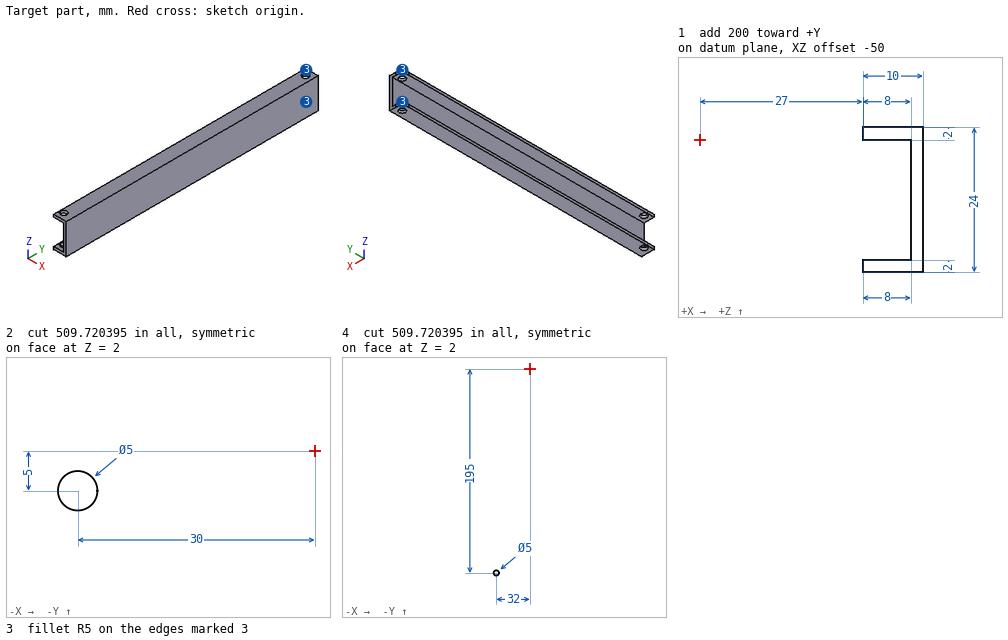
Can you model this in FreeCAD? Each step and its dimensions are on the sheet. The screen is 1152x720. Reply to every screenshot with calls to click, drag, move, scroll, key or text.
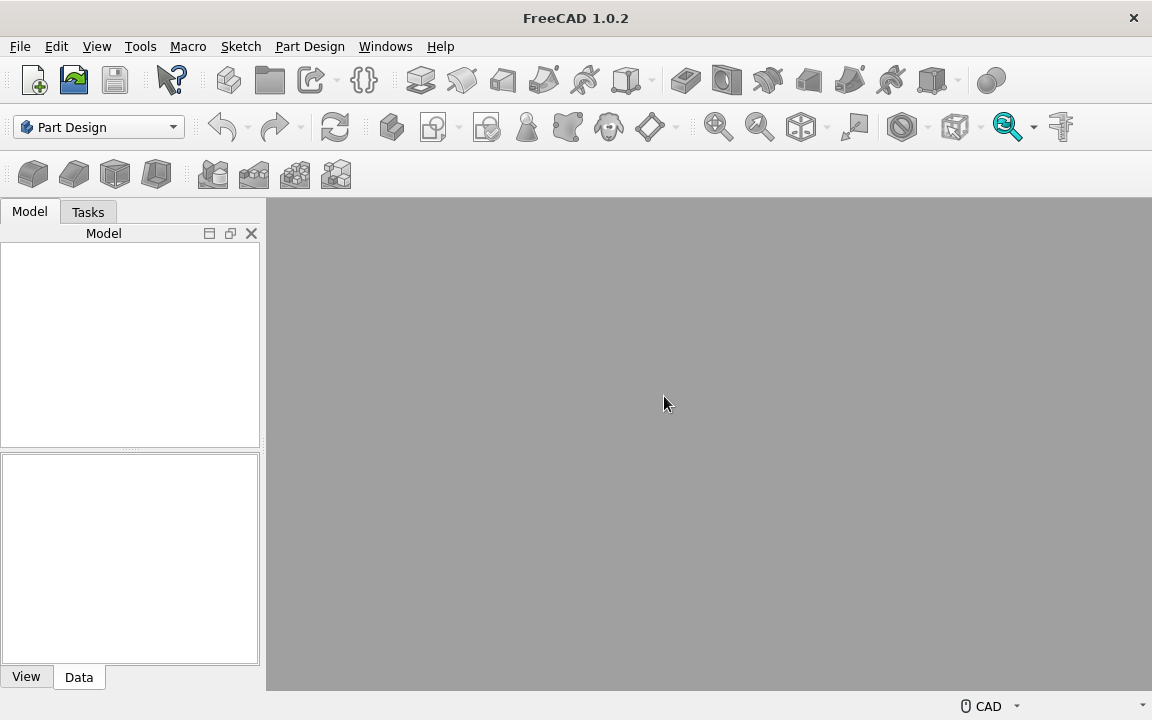
click(33, 80)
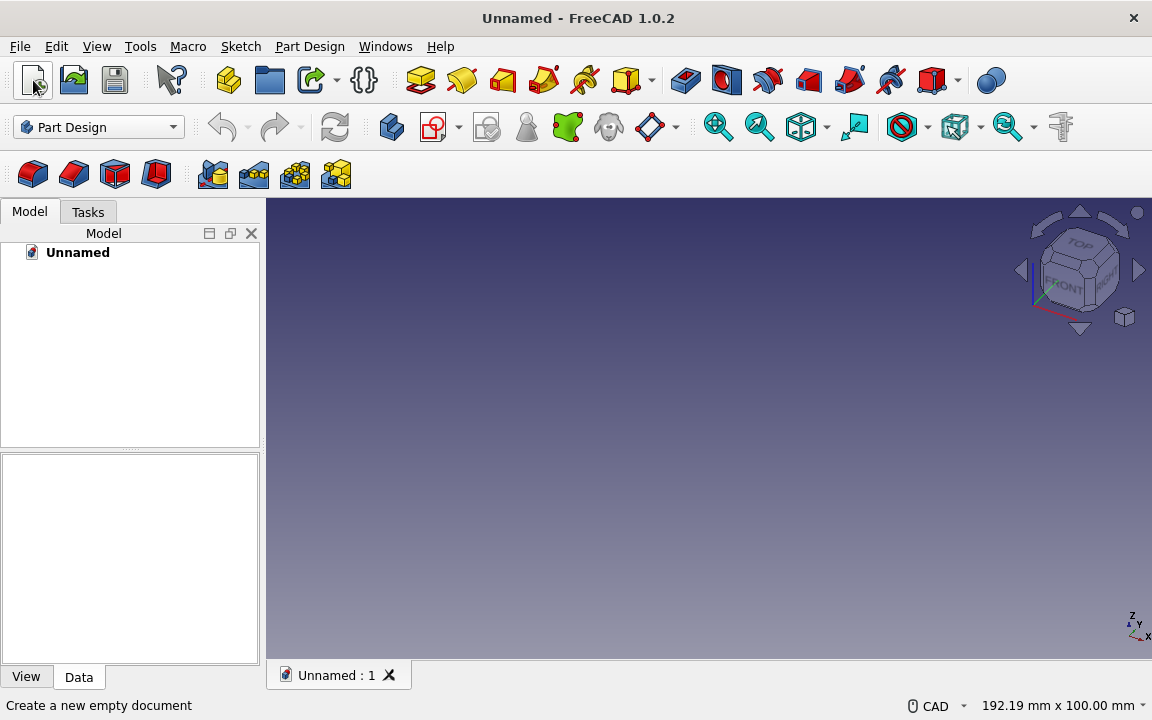
click(392, 128)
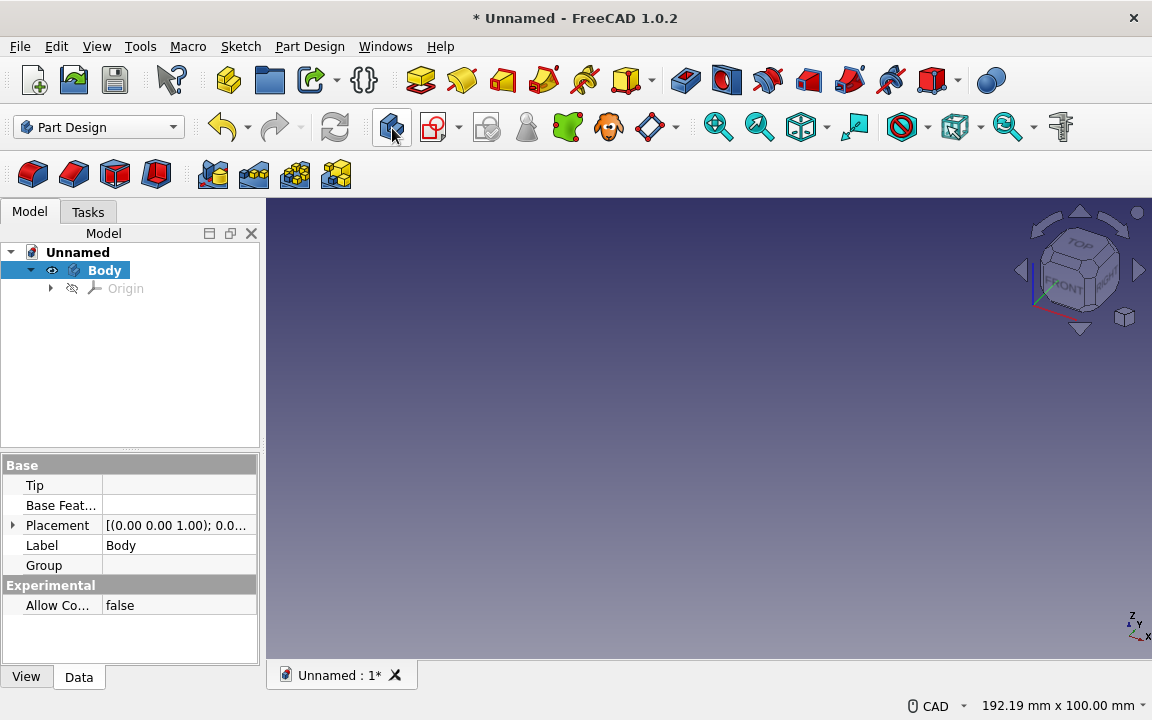
click(51, 288)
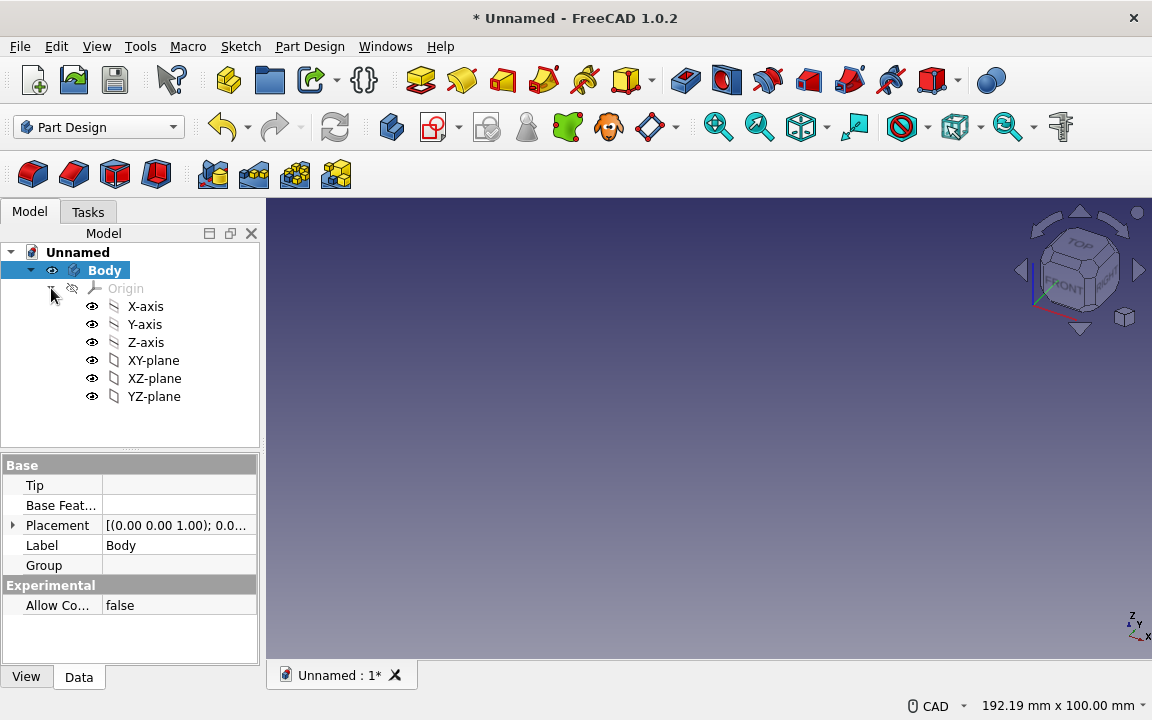
click(137, 378)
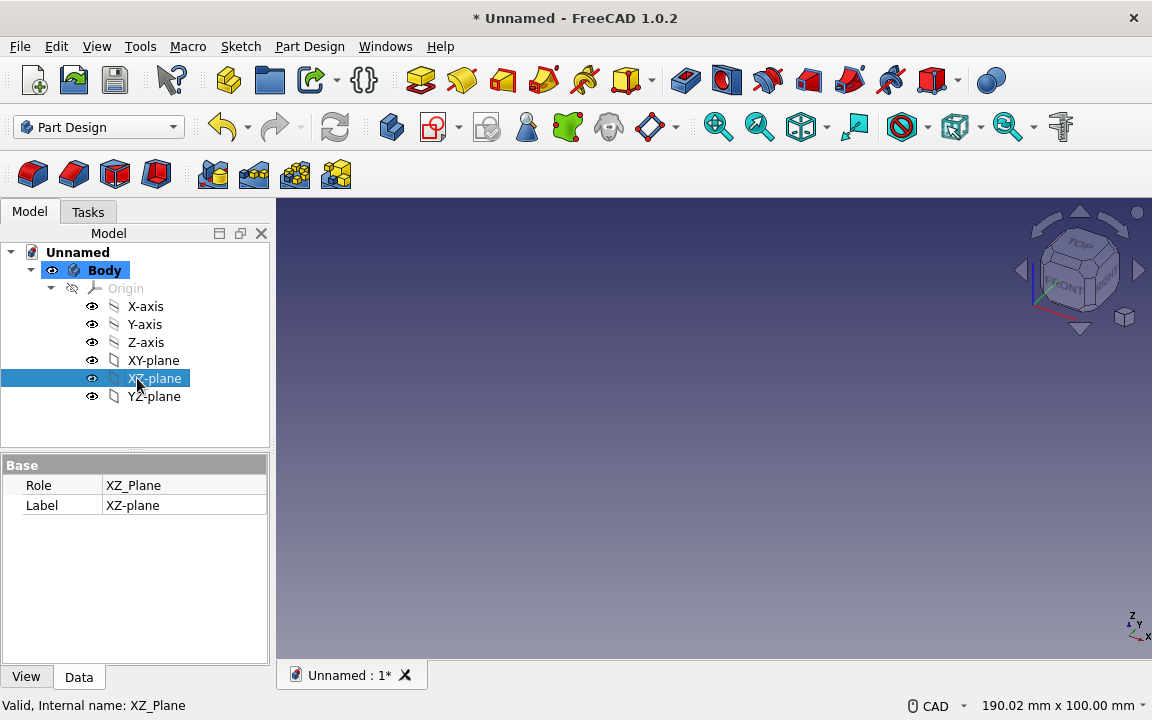
click(650, 128)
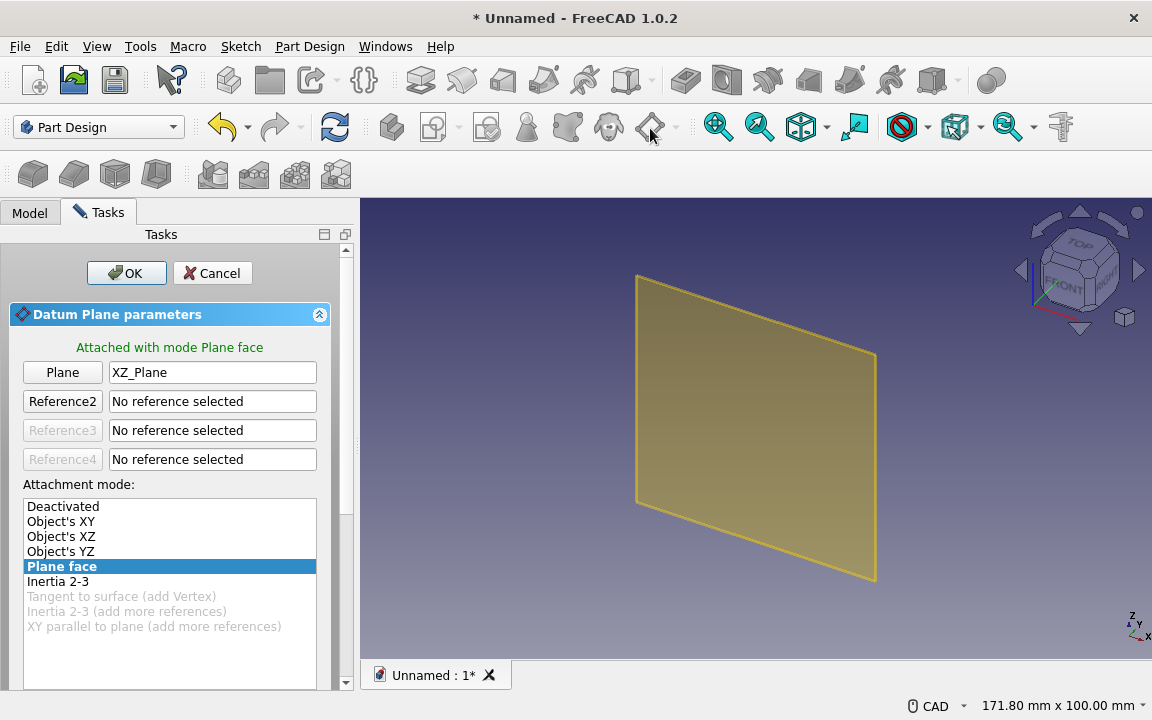
scroll(346, 467, down, 4)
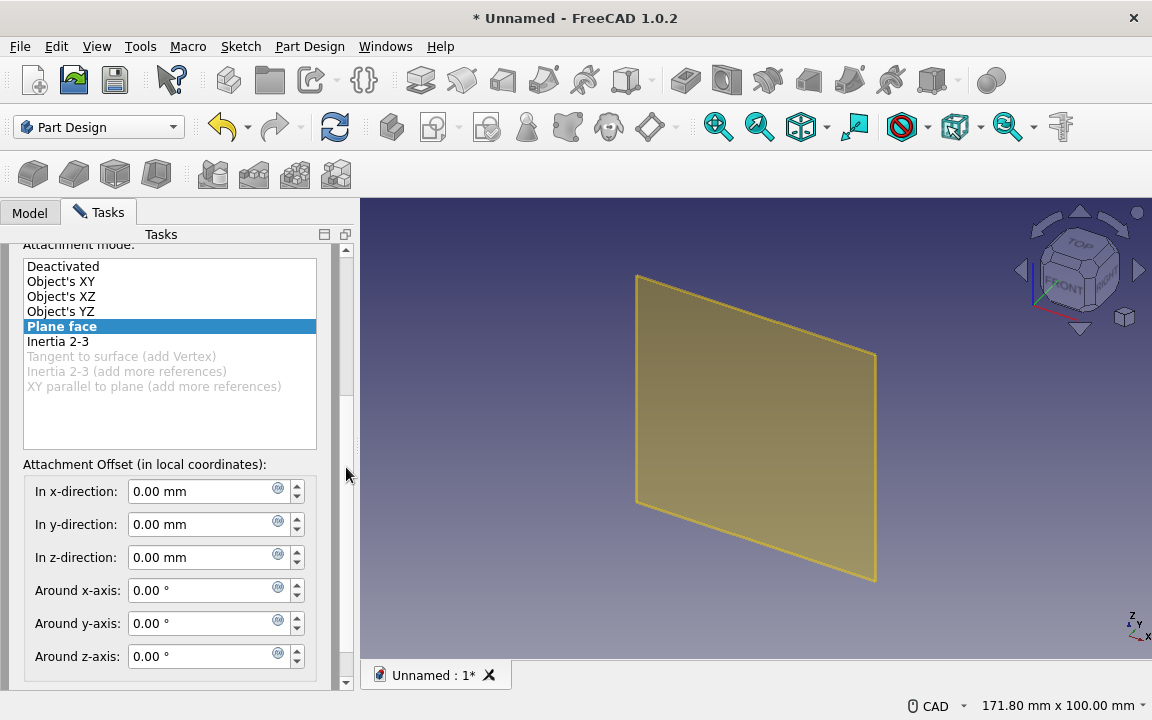
triple_click(210, 558)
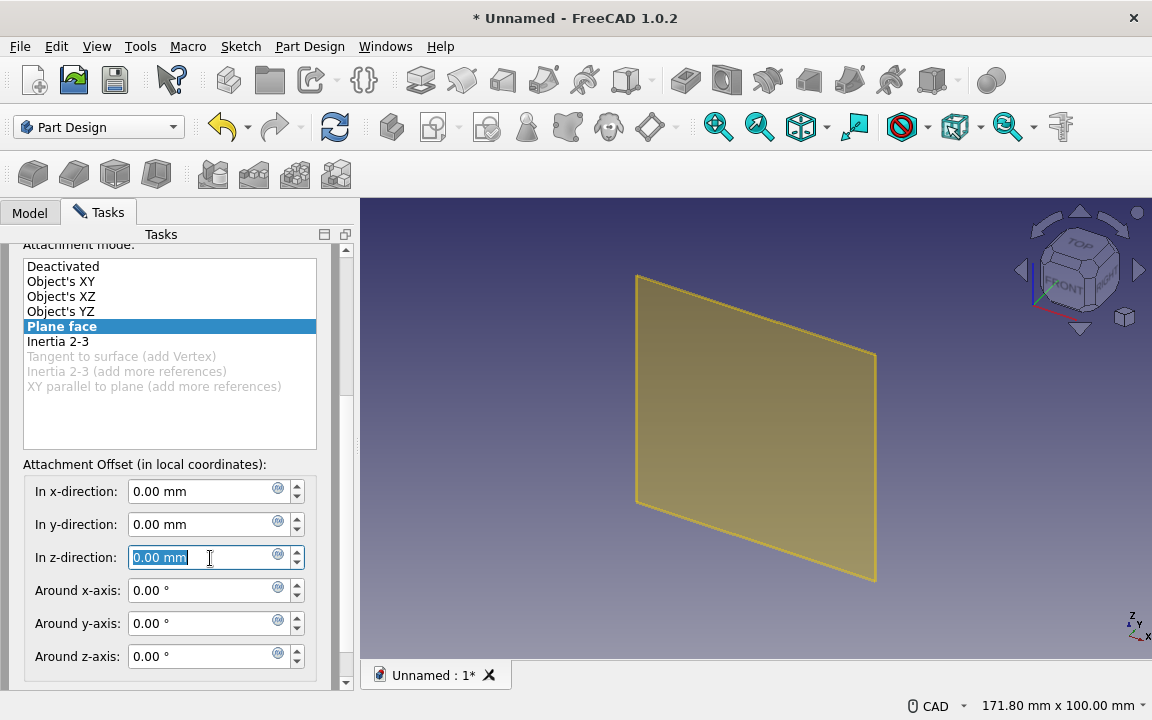
text(-50)
key(Tab)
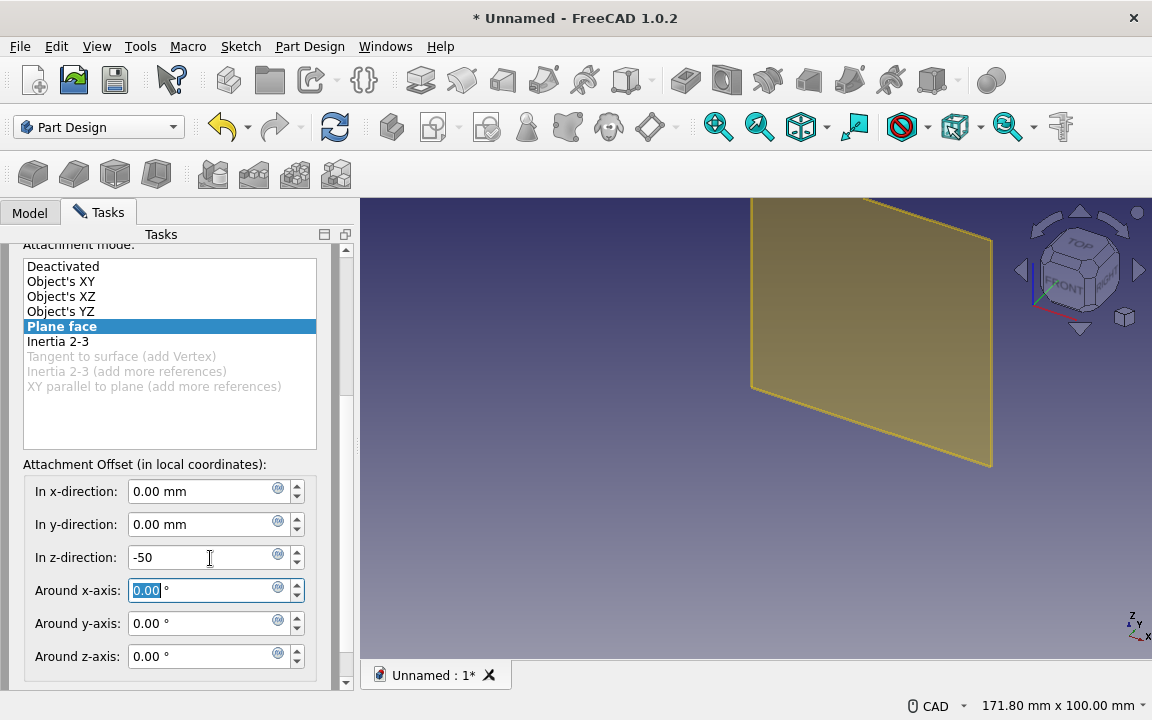
scroll(346, 467, up, 5)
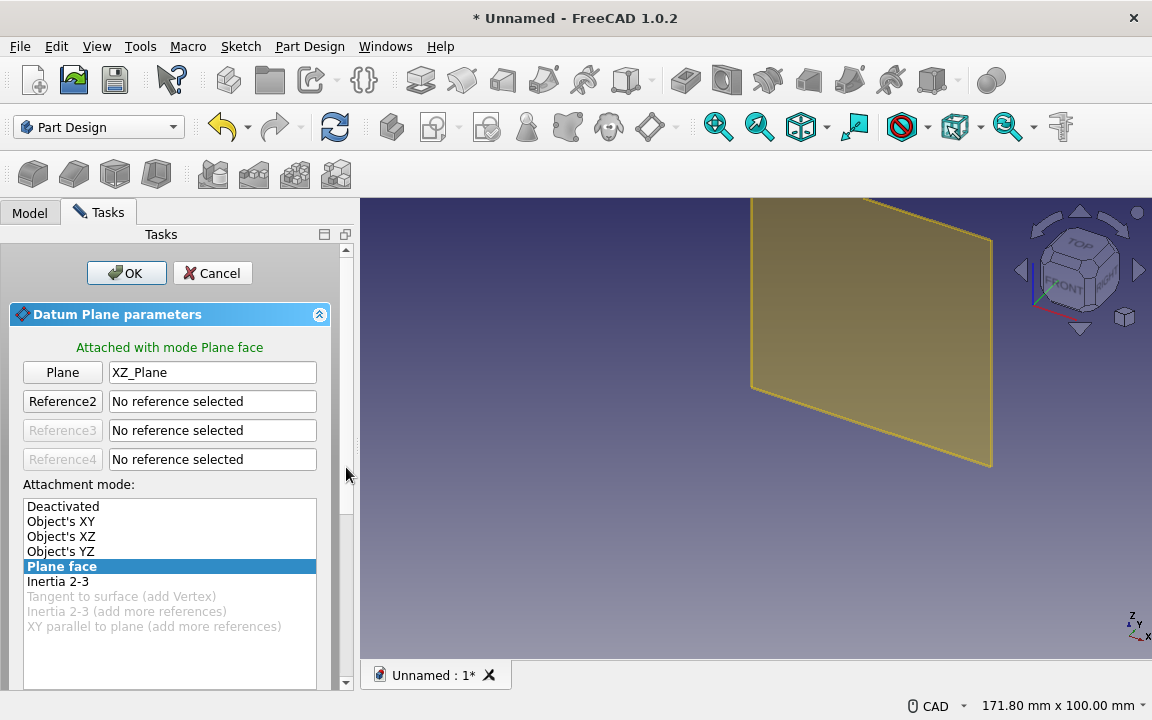
click(127, 273)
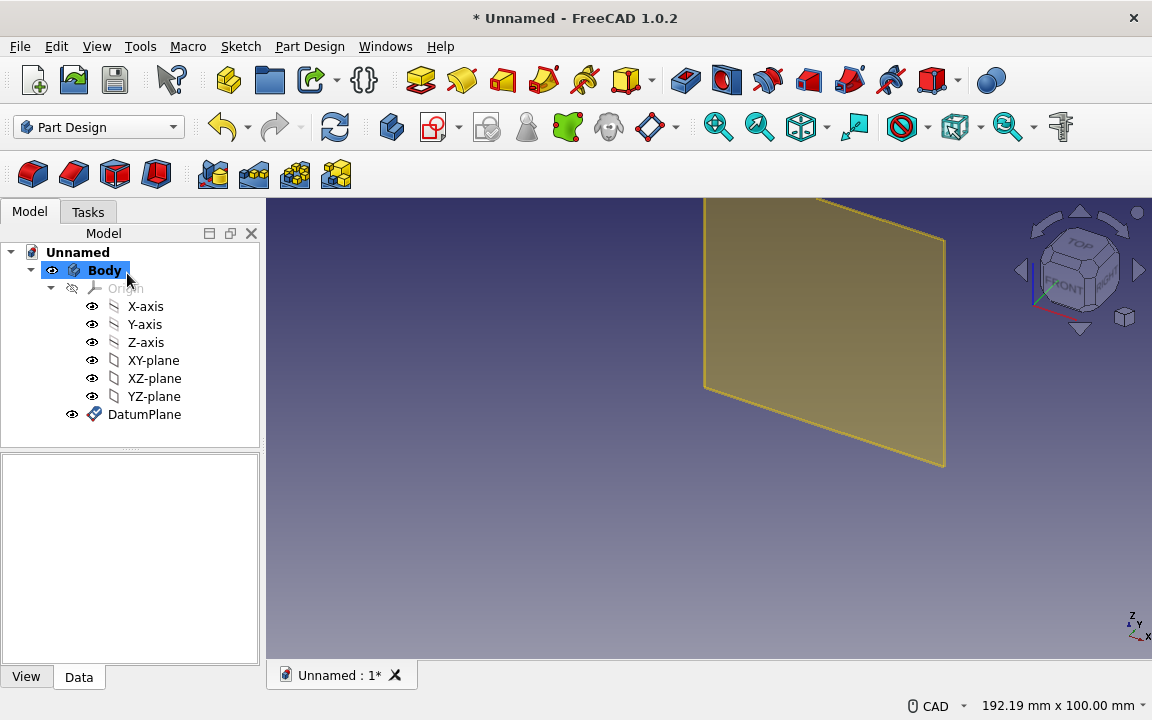
click(117, 414)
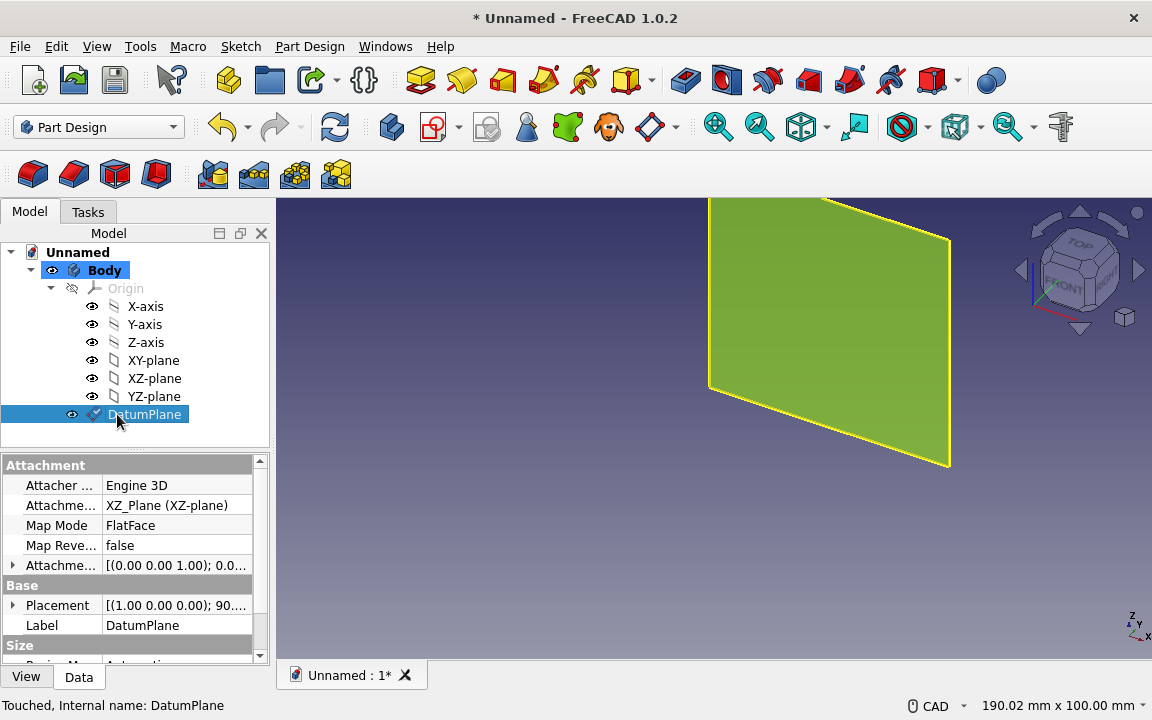
click(432, 128)